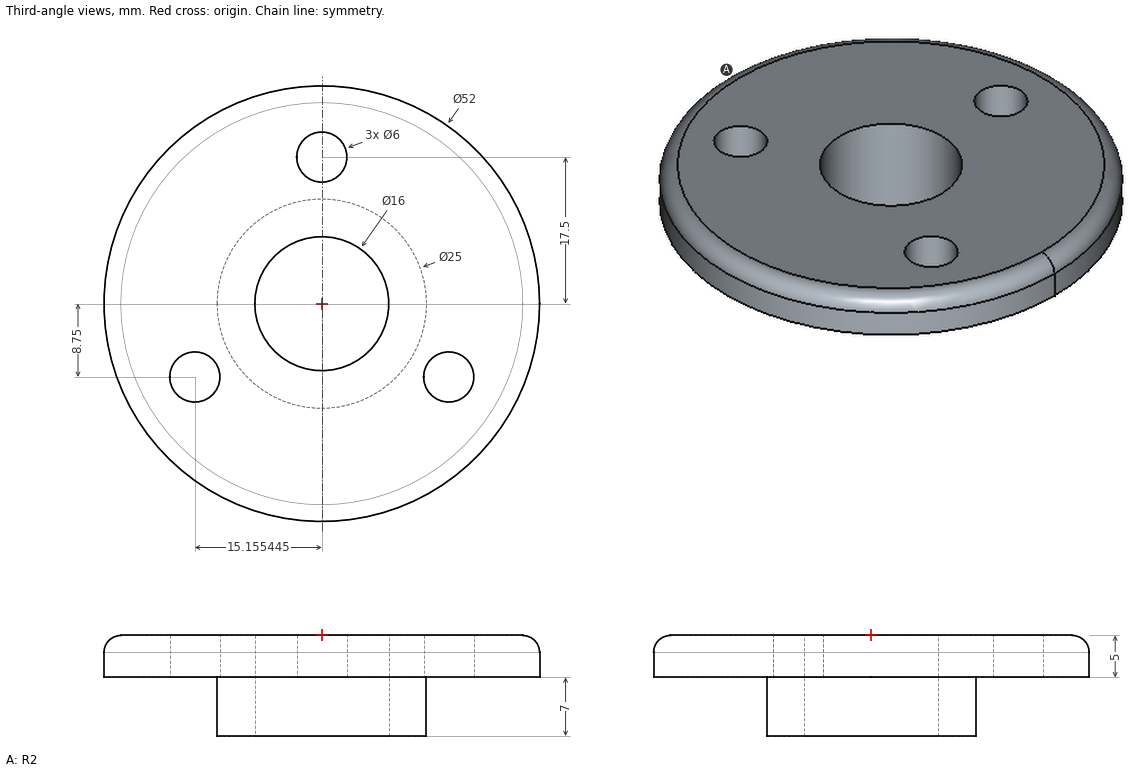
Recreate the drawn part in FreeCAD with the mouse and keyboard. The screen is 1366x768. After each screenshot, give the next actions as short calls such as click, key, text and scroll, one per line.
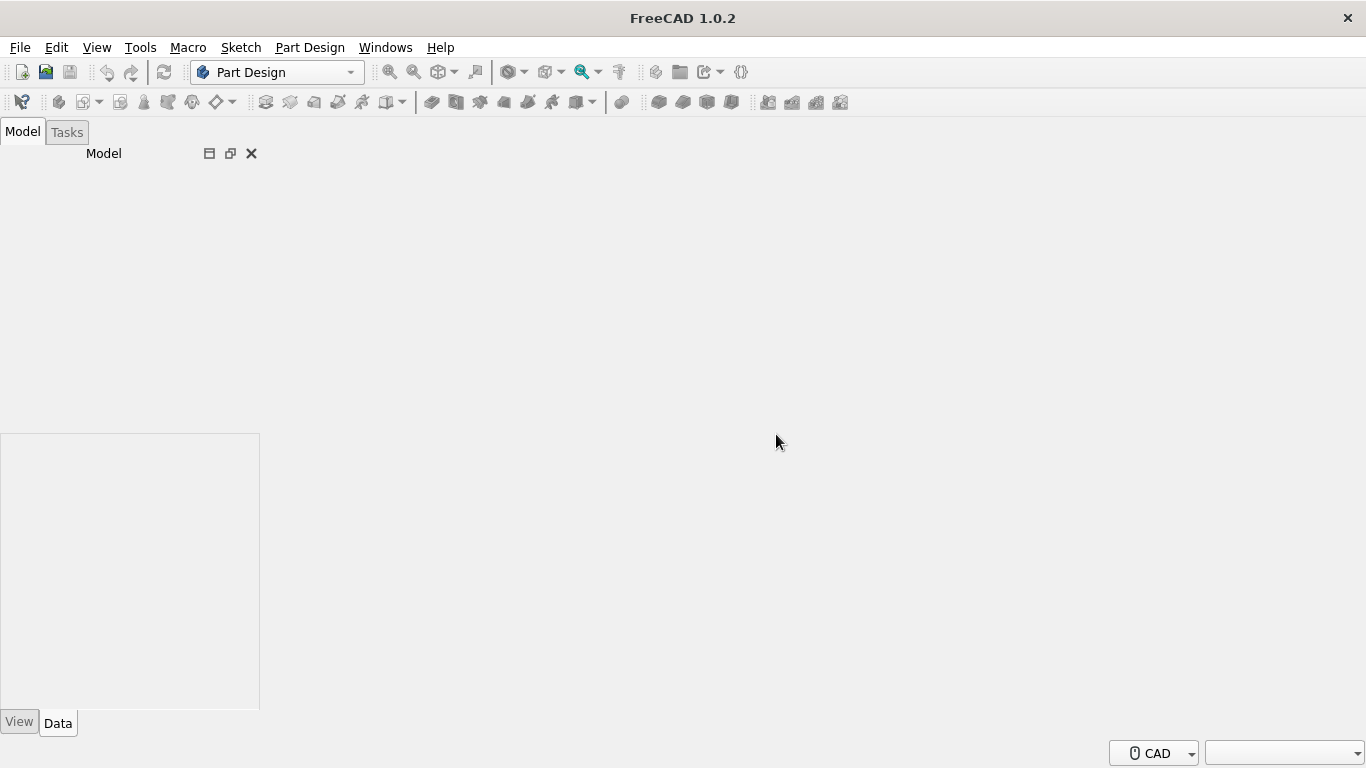
click(22, 72)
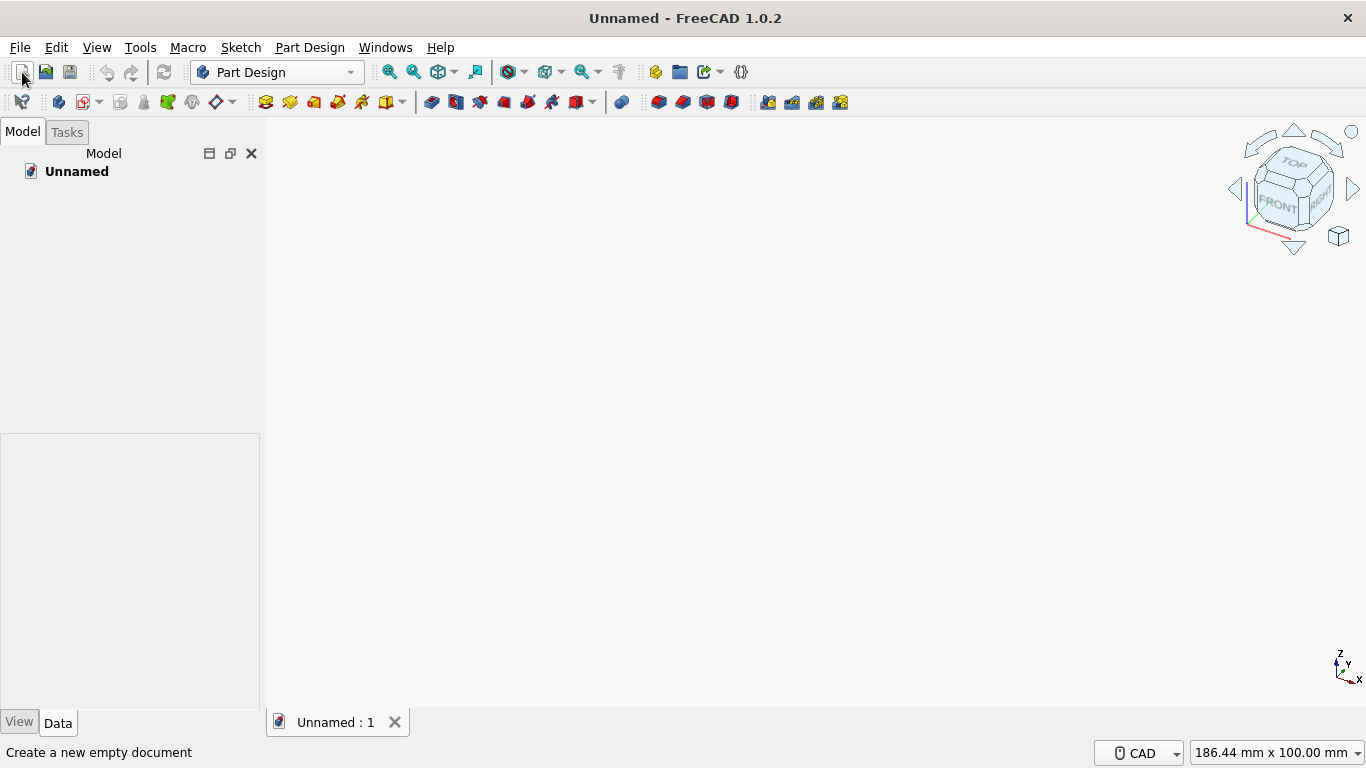
click(84, 102)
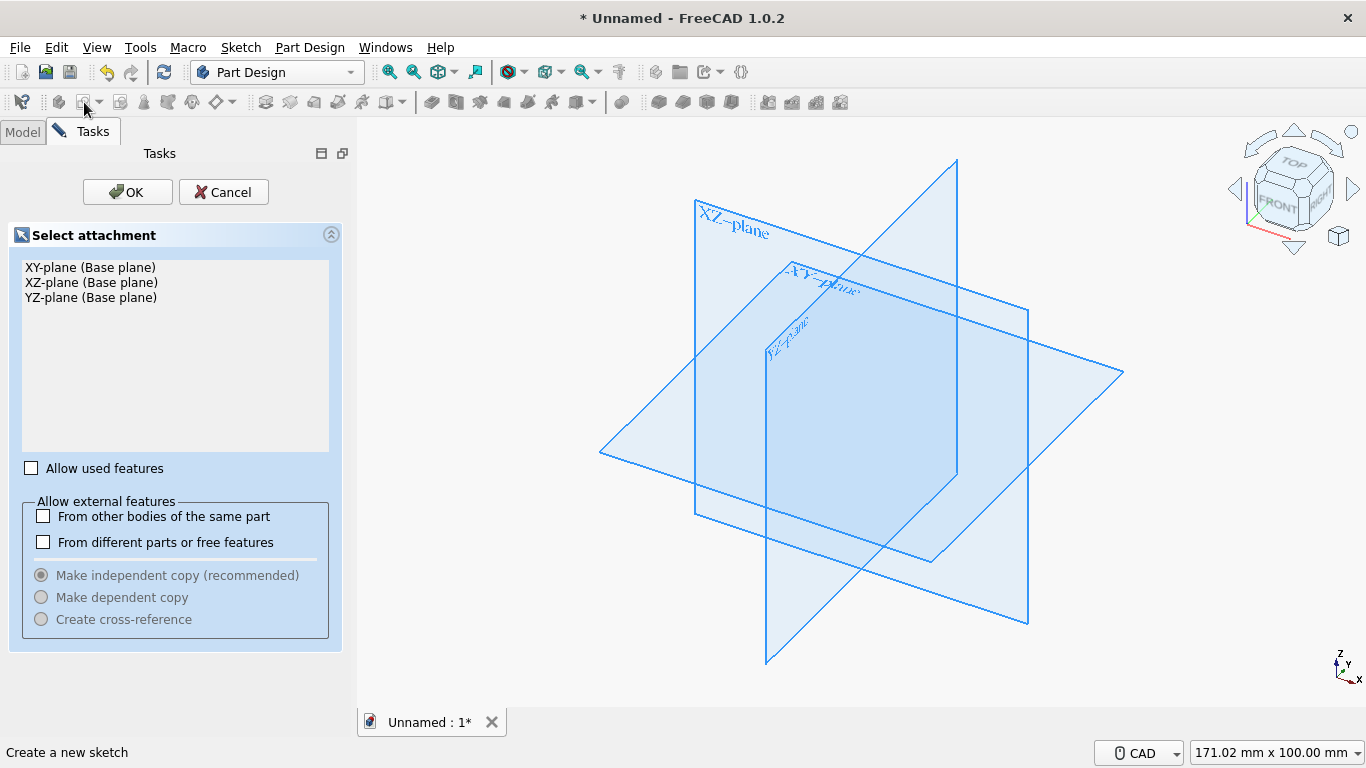
click(82, 268)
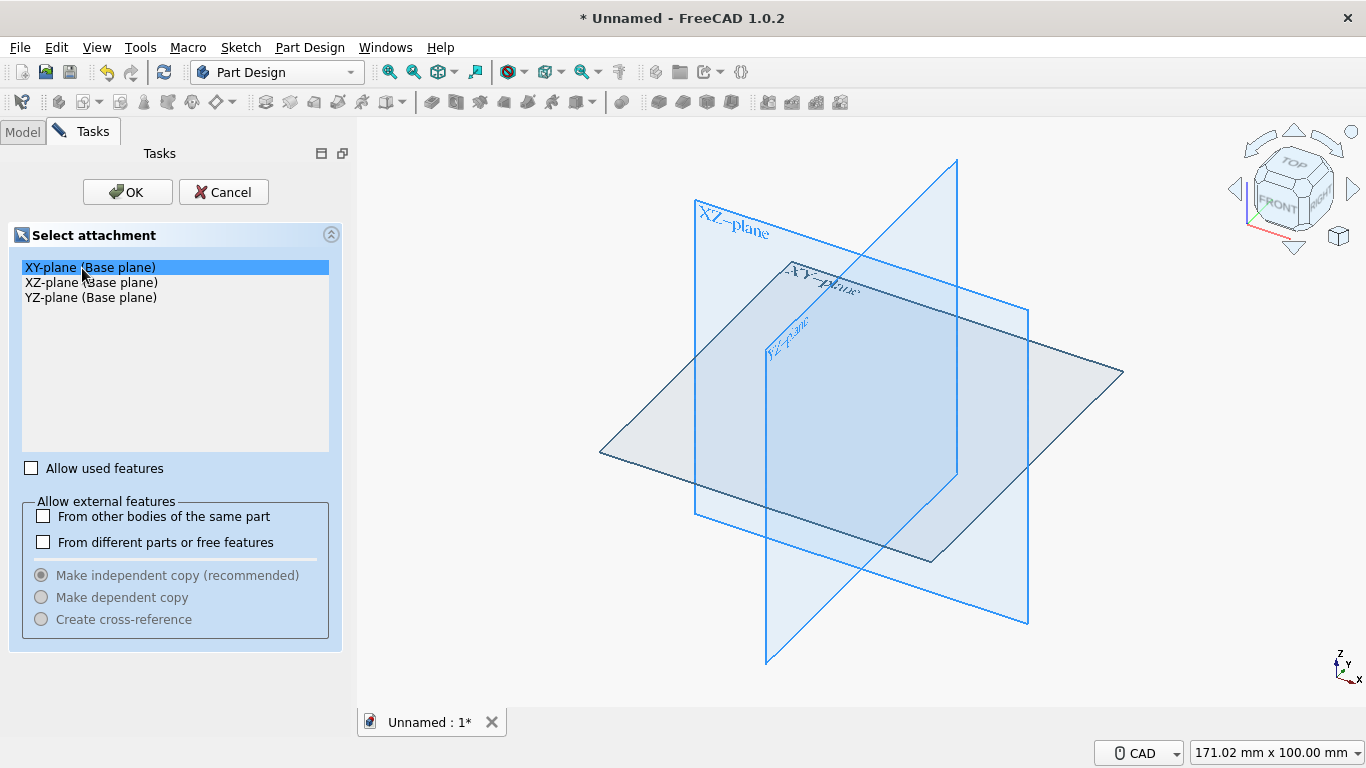
click(128, 192)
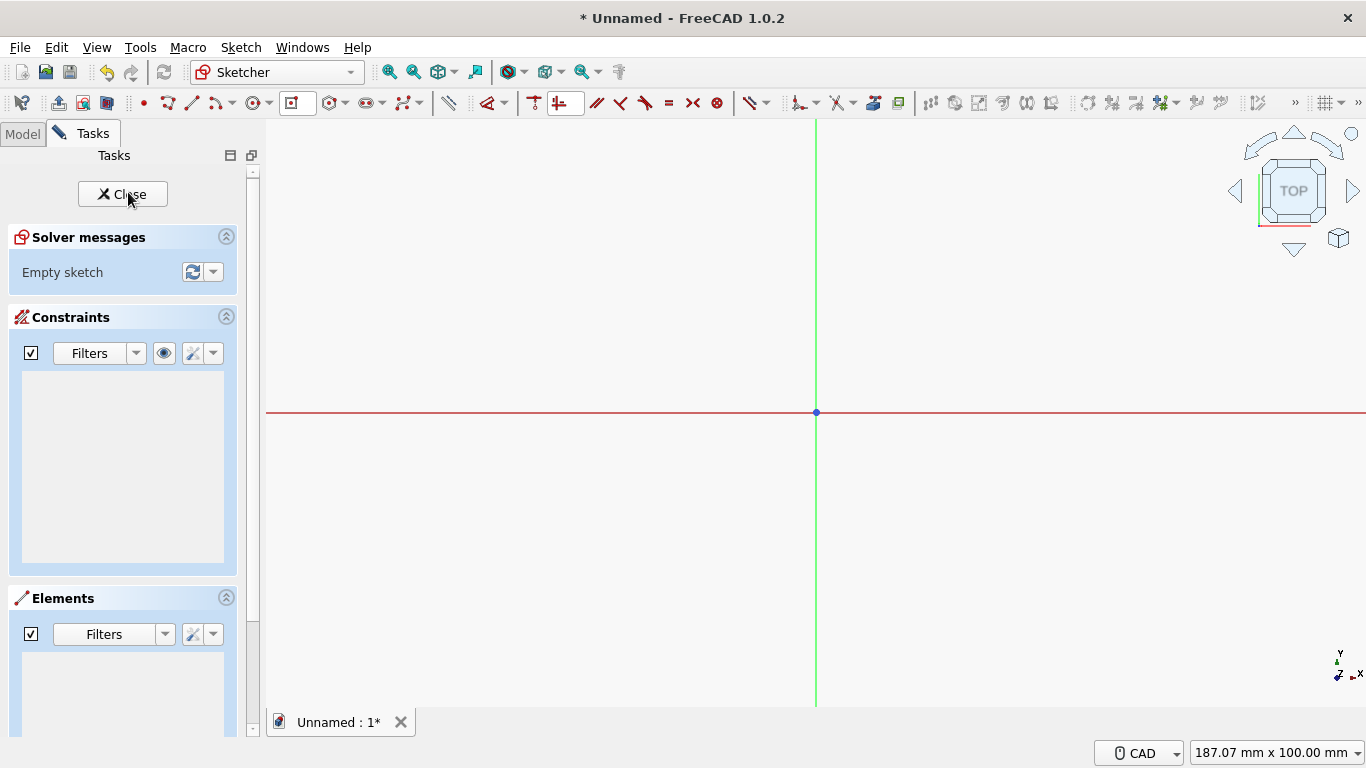
click(254, 104)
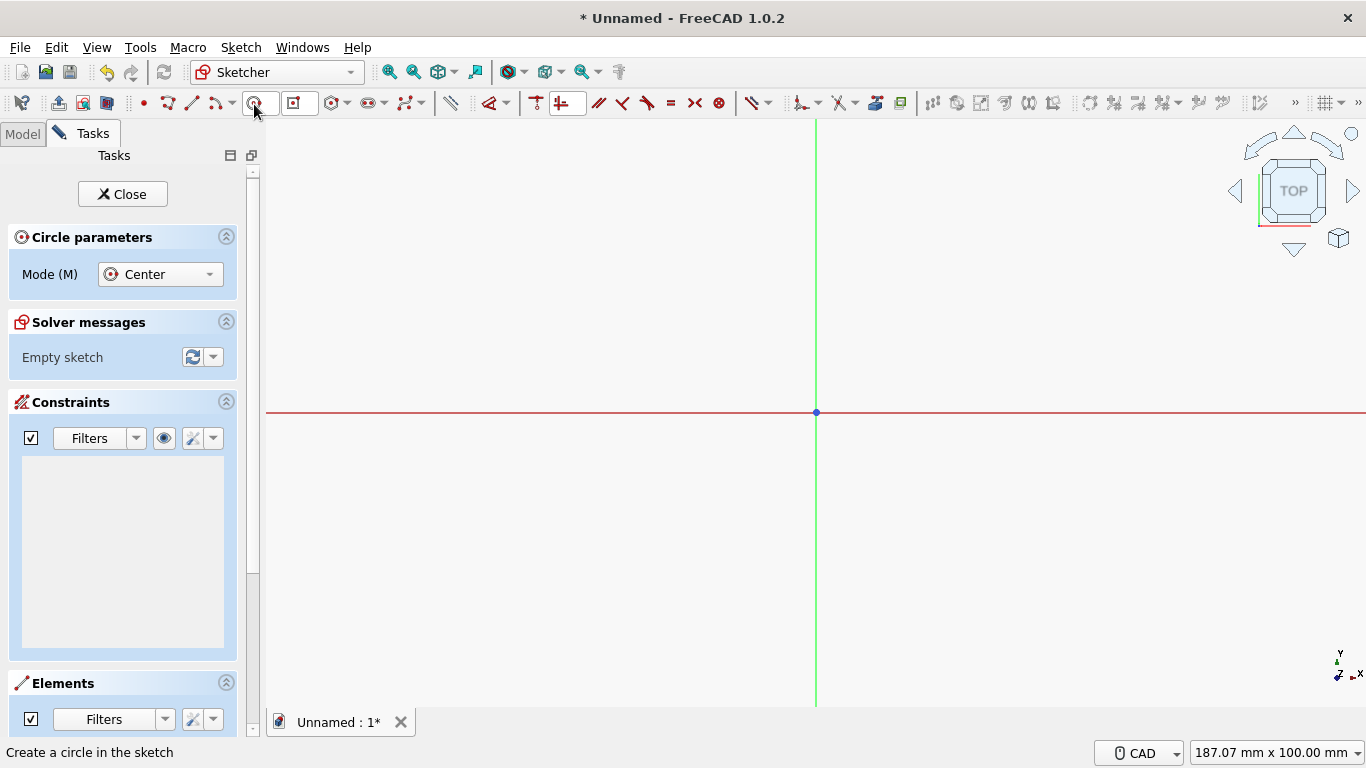
click(816, 413)
move(924, 305)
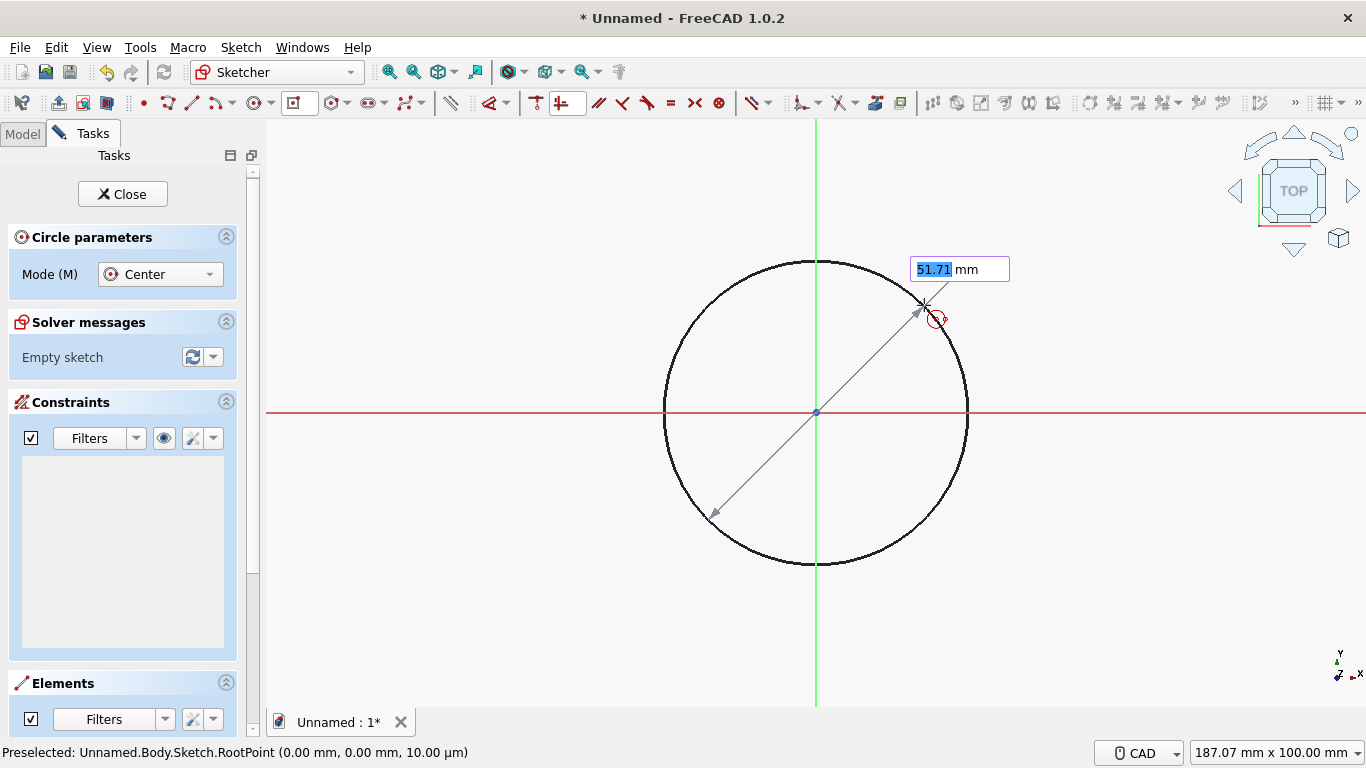
text(52)
key(Return)
key(Escape)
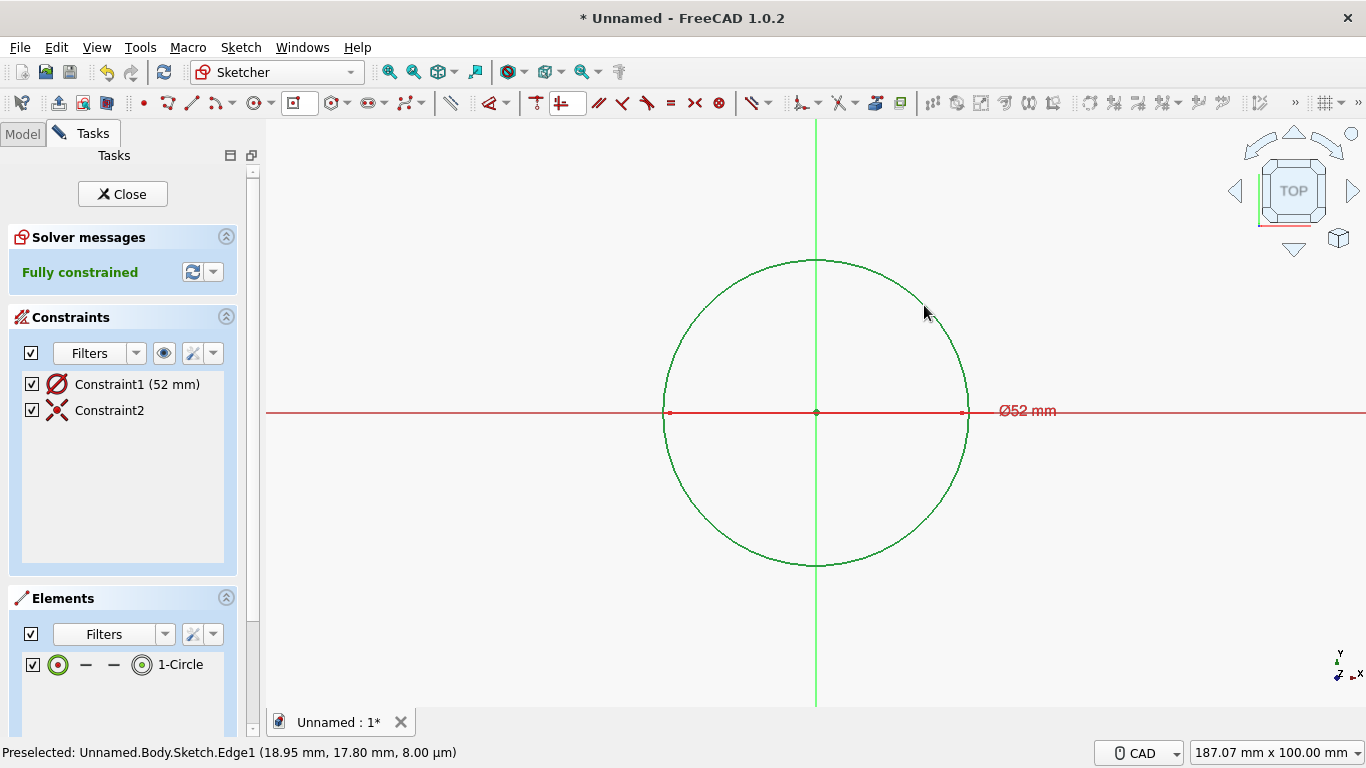
click(123, 194)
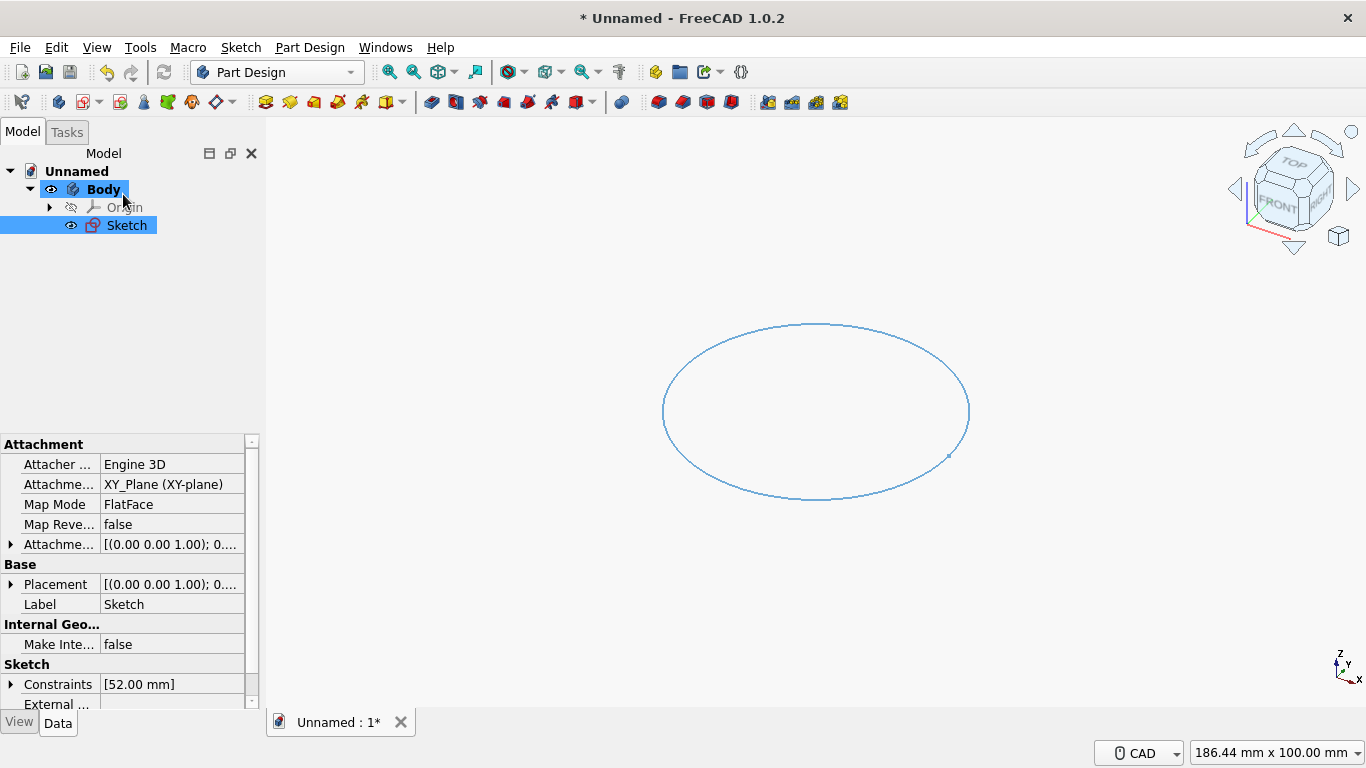
click(266, 102)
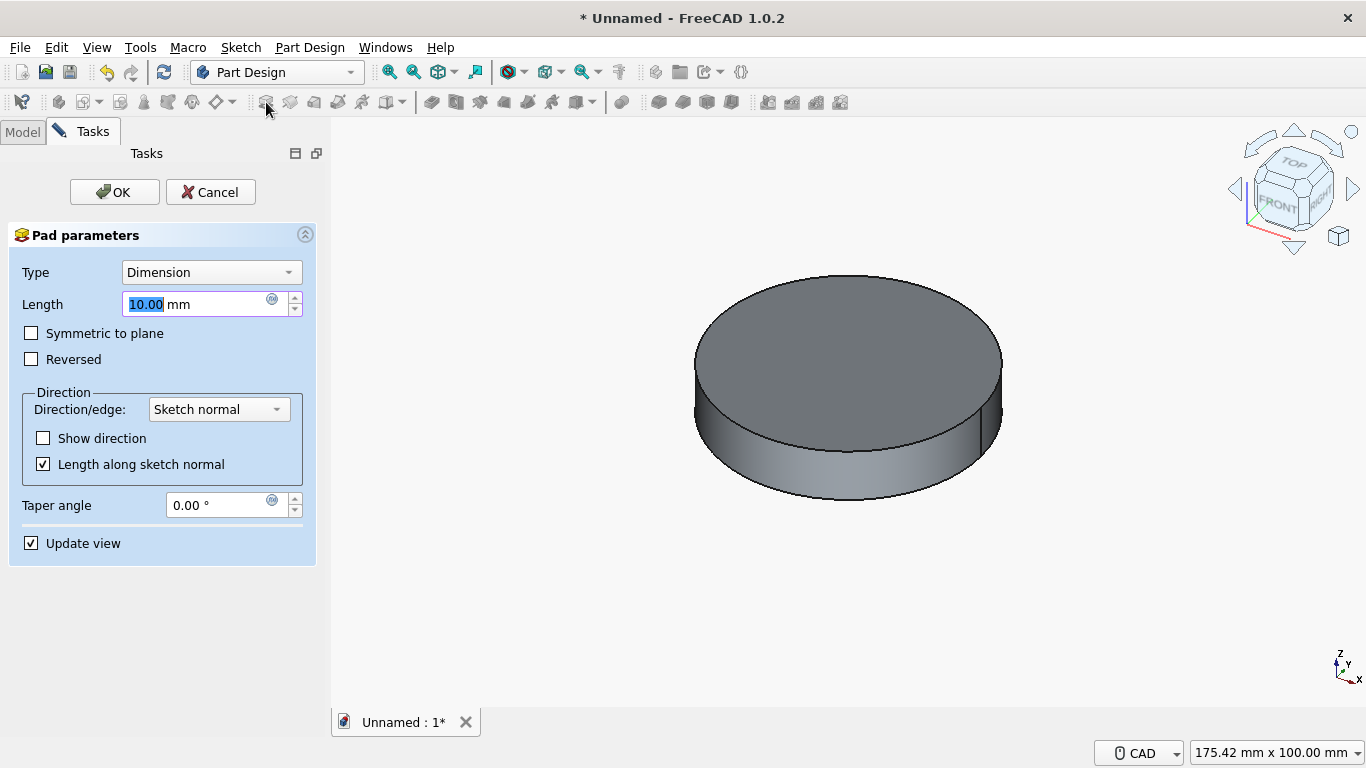
text(5)
key(Tab)